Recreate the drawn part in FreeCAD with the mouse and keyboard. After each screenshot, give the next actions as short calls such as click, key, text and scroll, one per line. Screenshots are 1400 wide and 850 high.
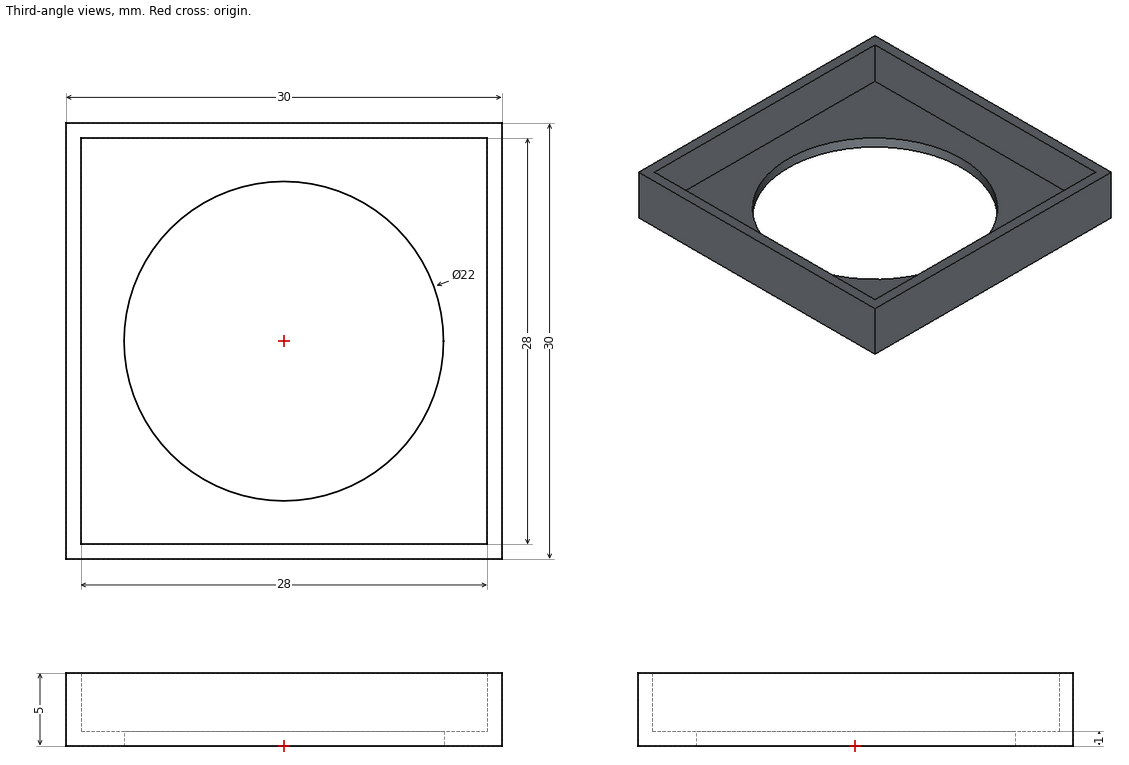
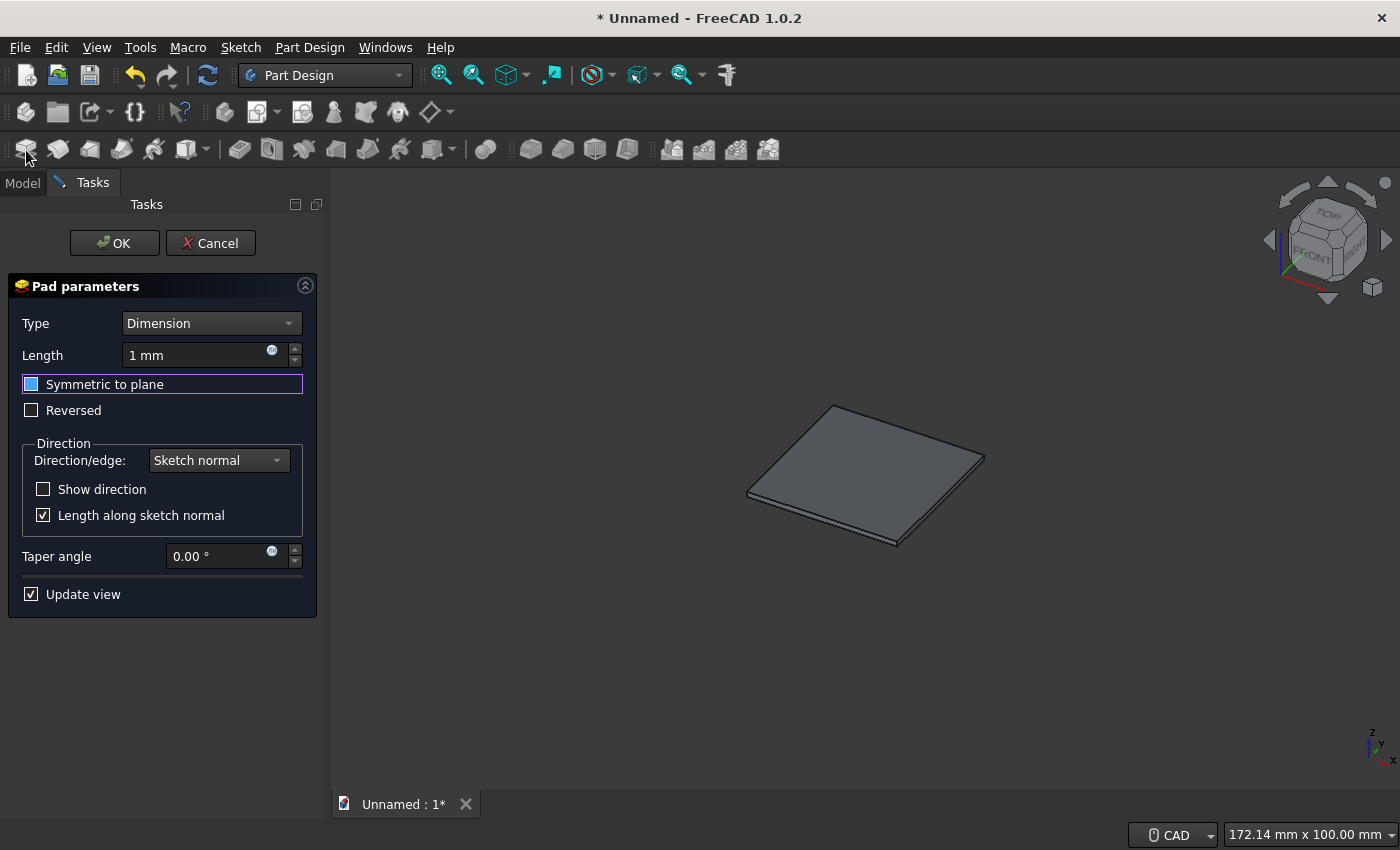
click(115, 243)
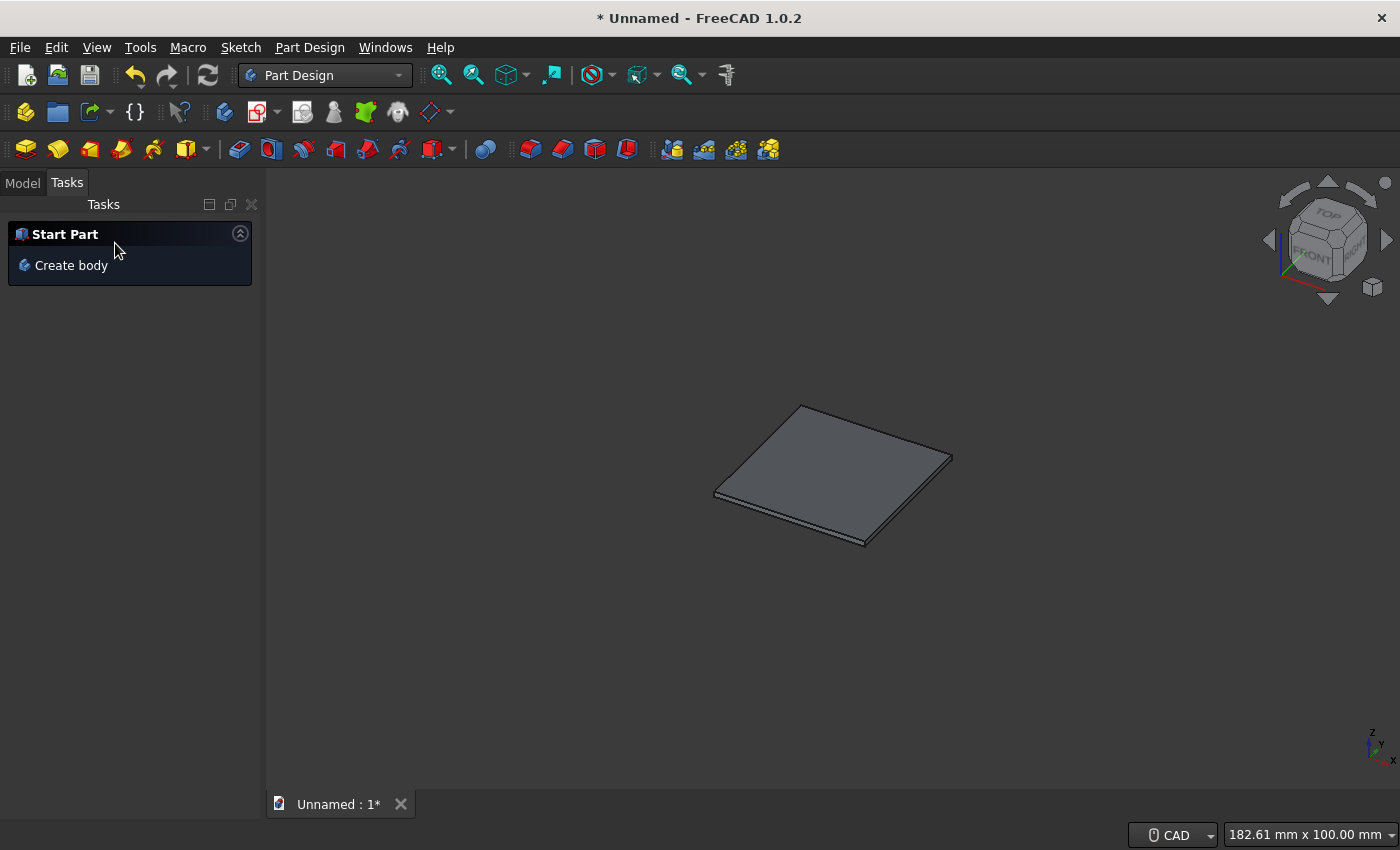
click(442, 76)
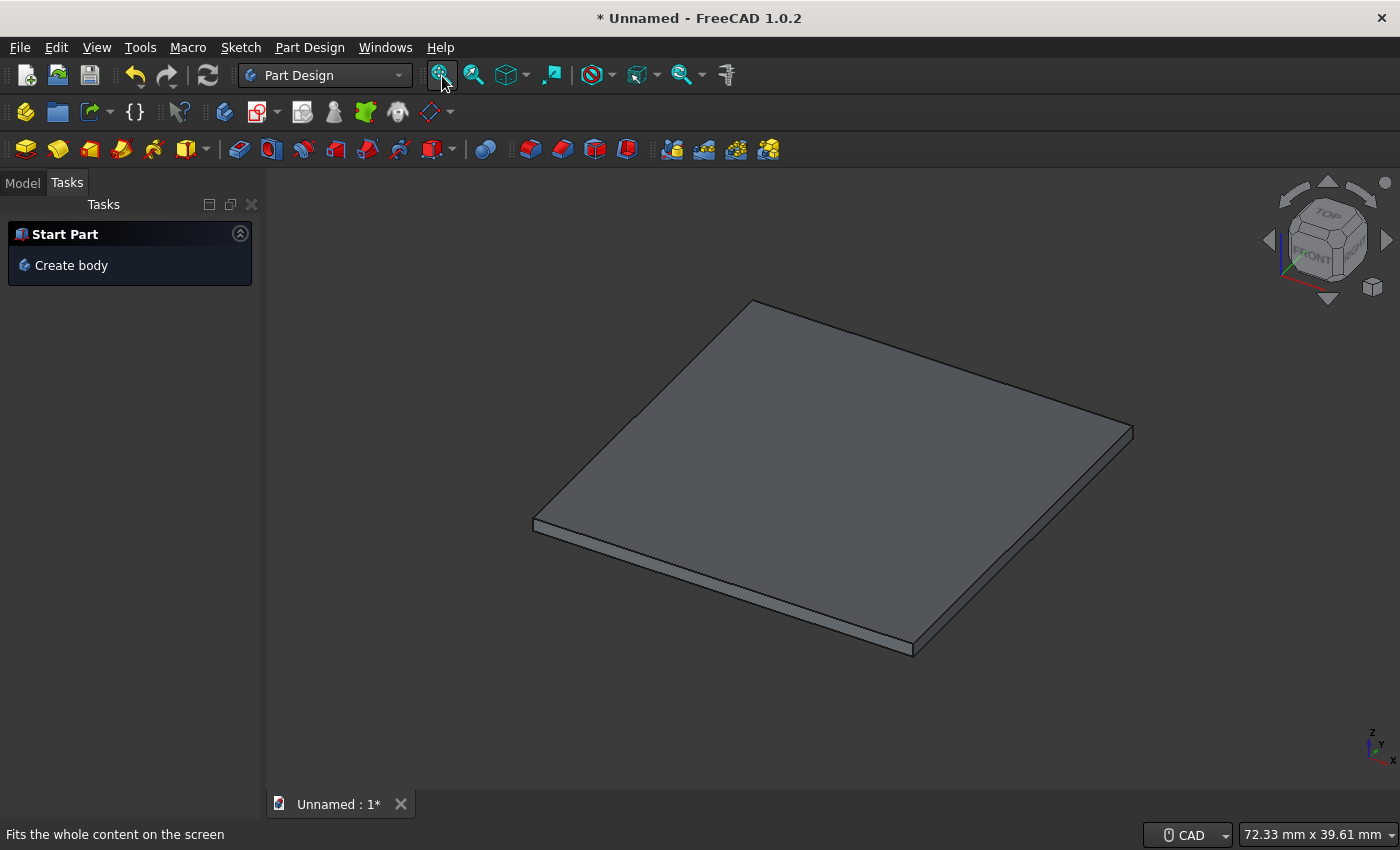
key(5)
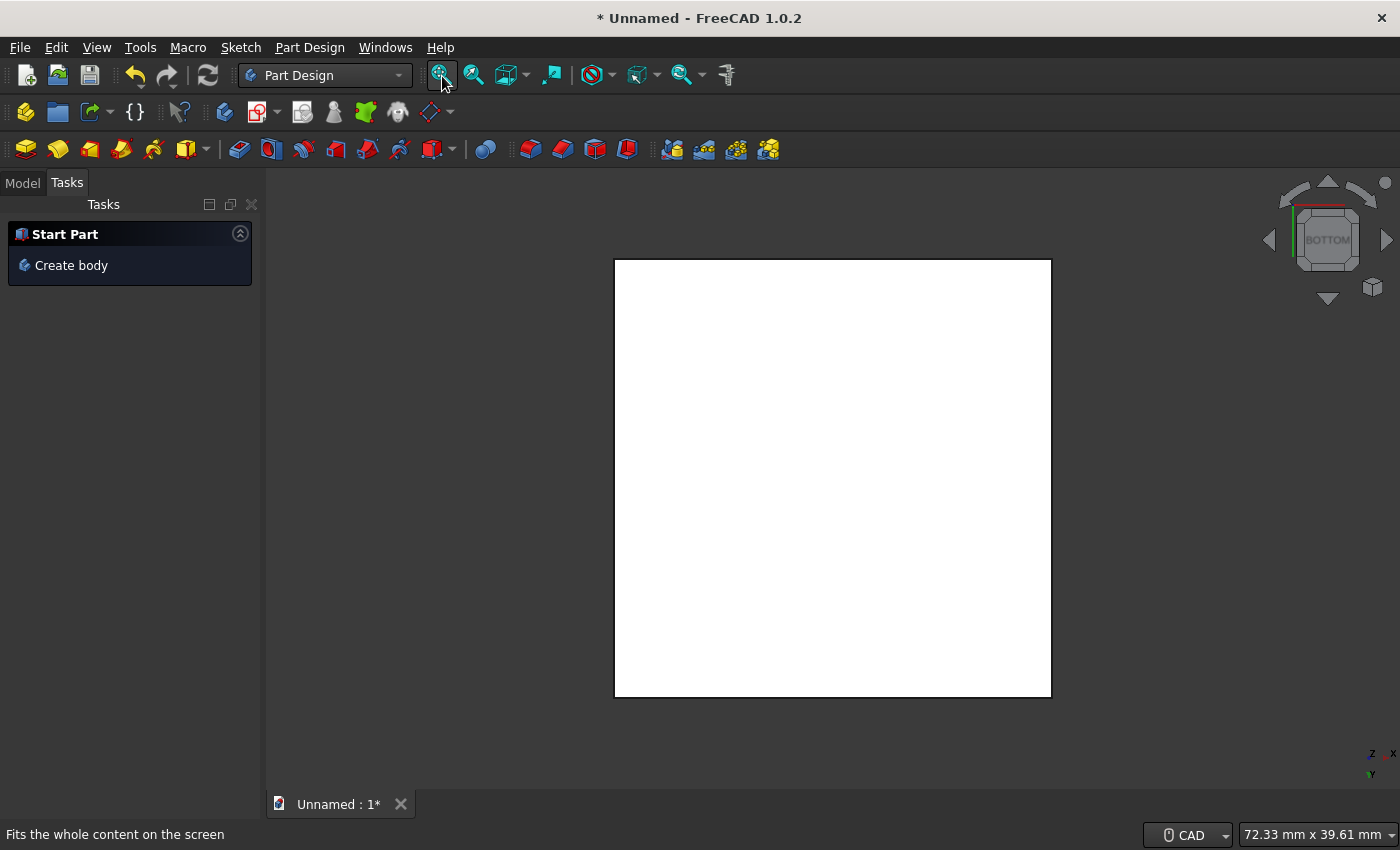
click(833, 477)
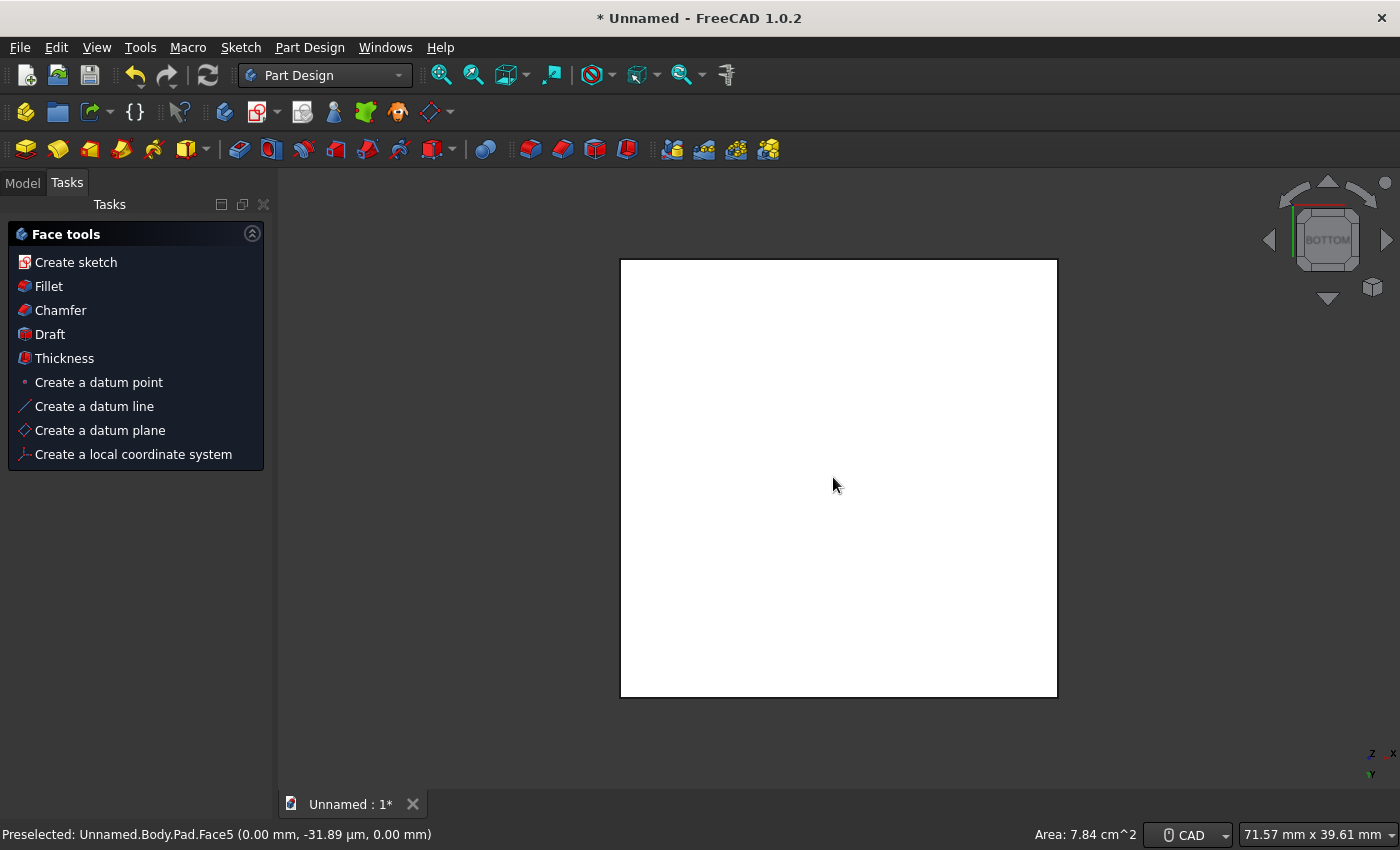
click(258, 112)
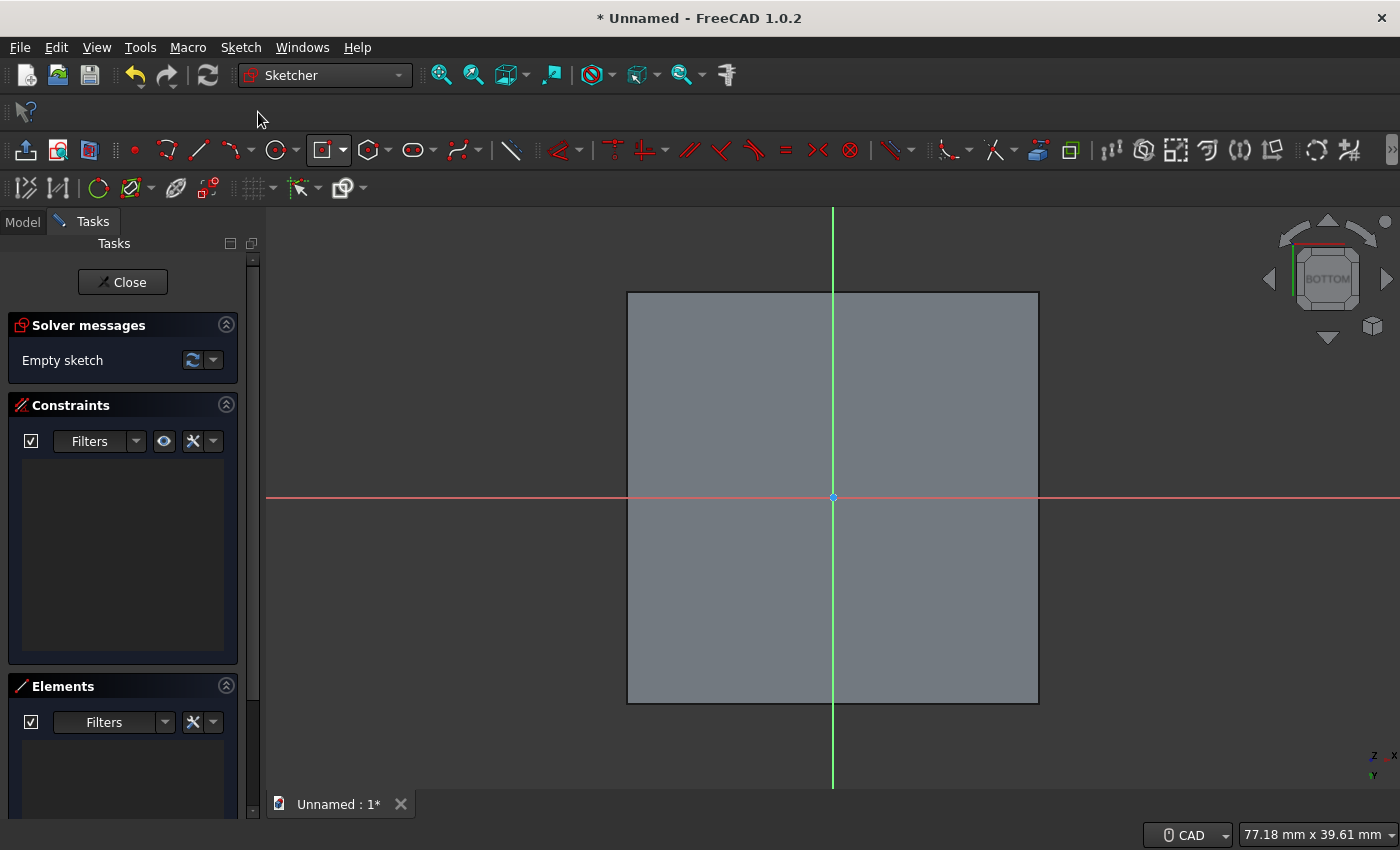
click(322, 150)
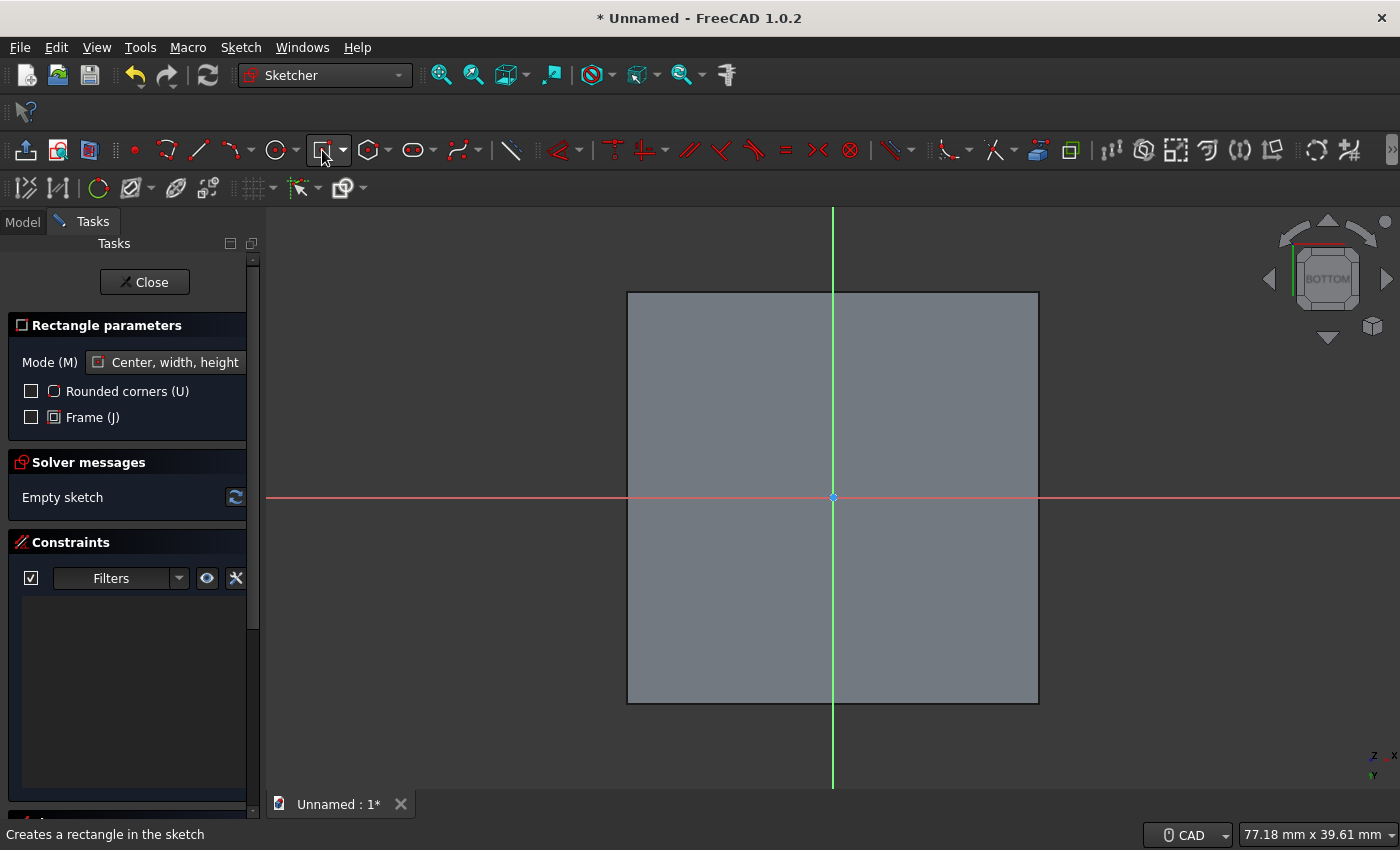
click(833, 498)
click(1053, 278)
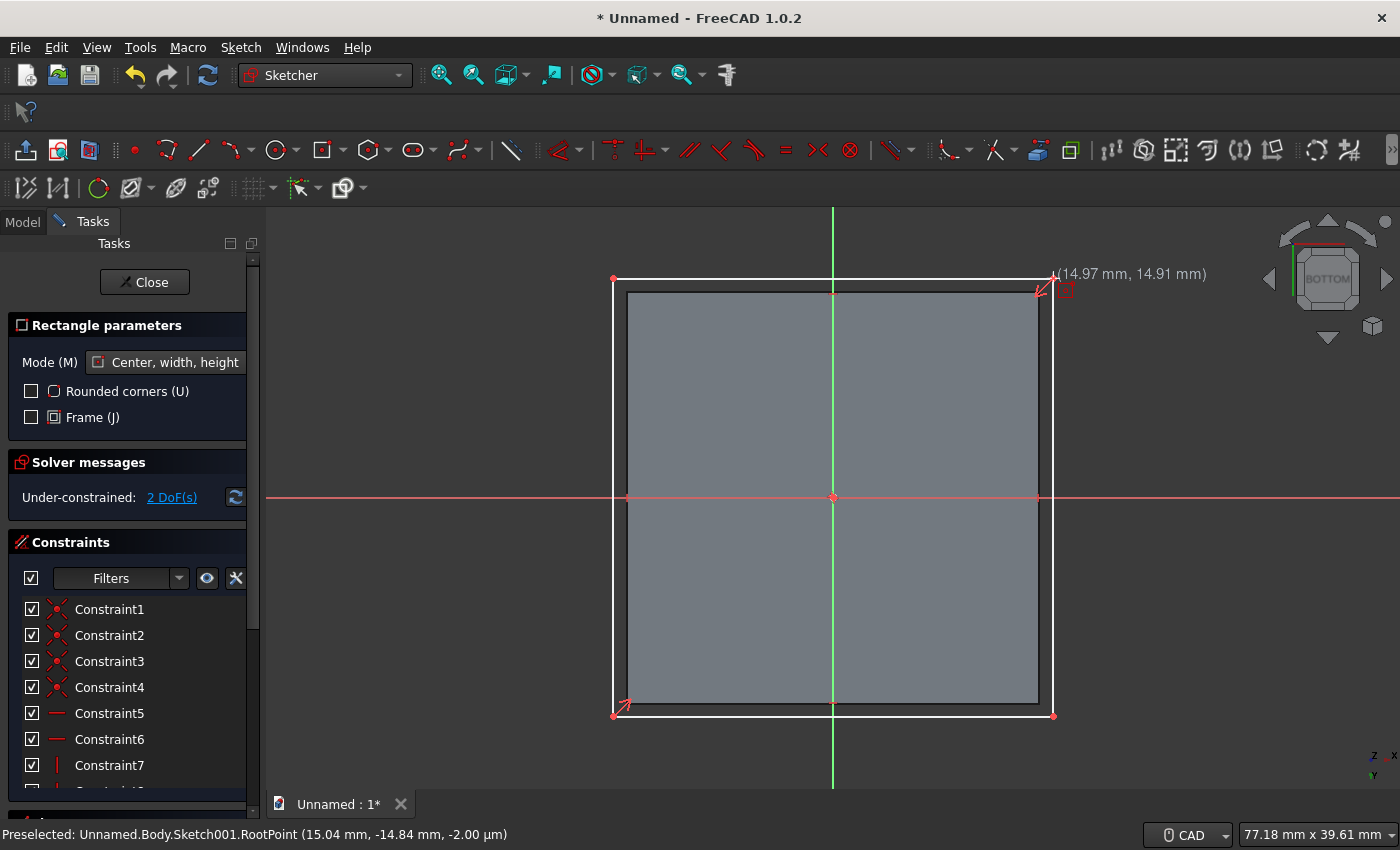
click(833, 498)
click(1039, 292)
key(Escape)